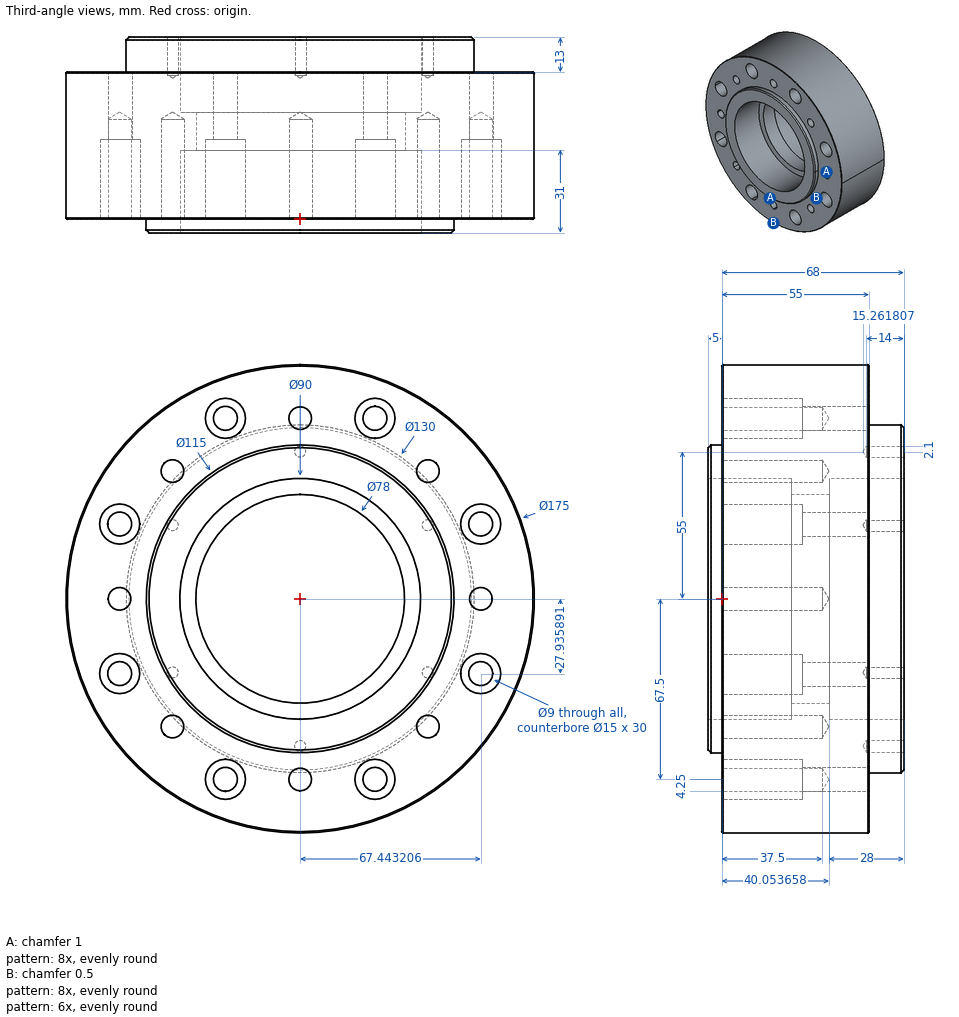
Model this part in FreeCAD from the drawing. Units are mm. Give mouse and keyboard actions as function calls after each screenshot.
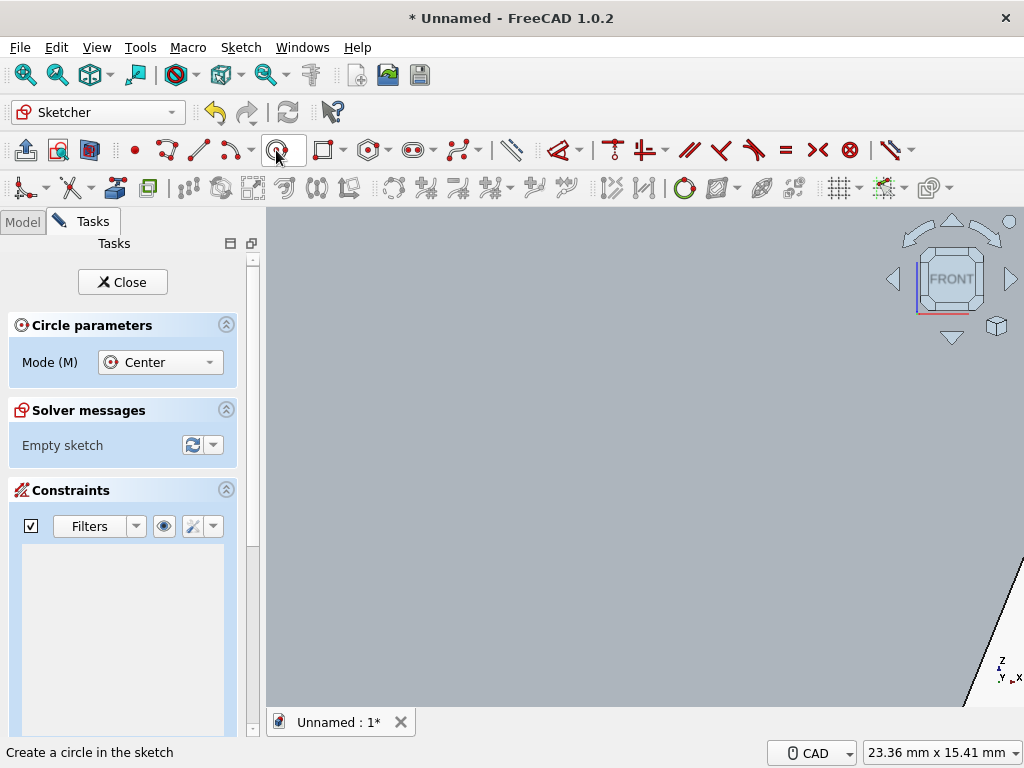
click(568, 440)
click(672, 337)
key(Escape)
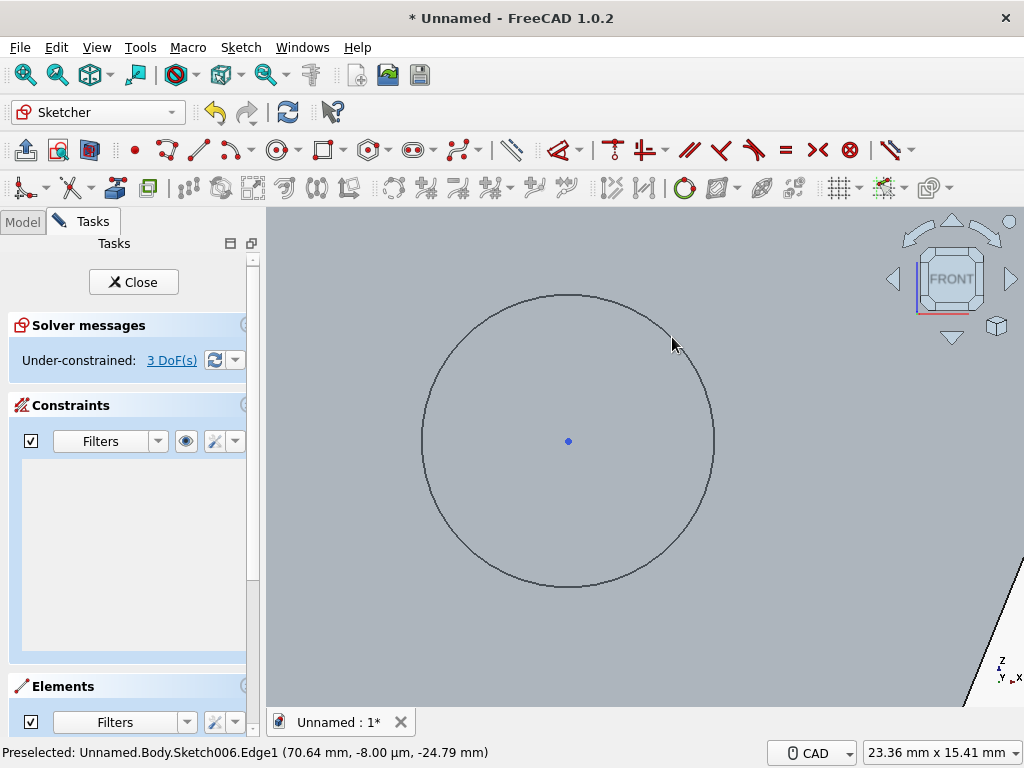
click(558, 150)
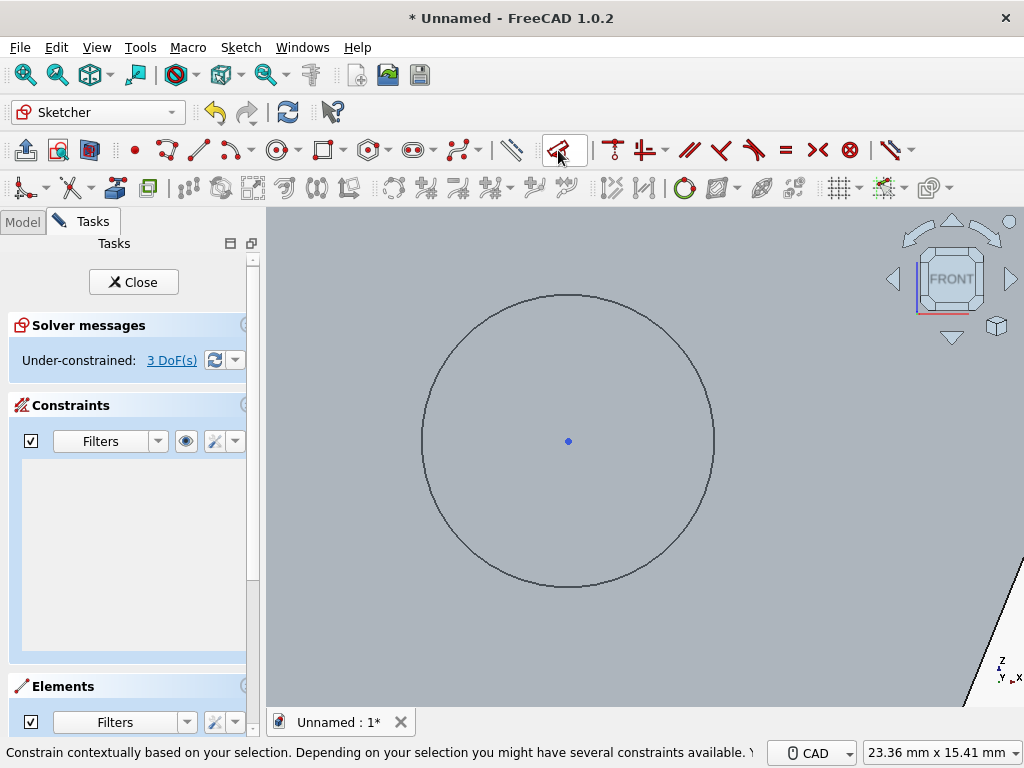
click(671, 337)
click(694, 314)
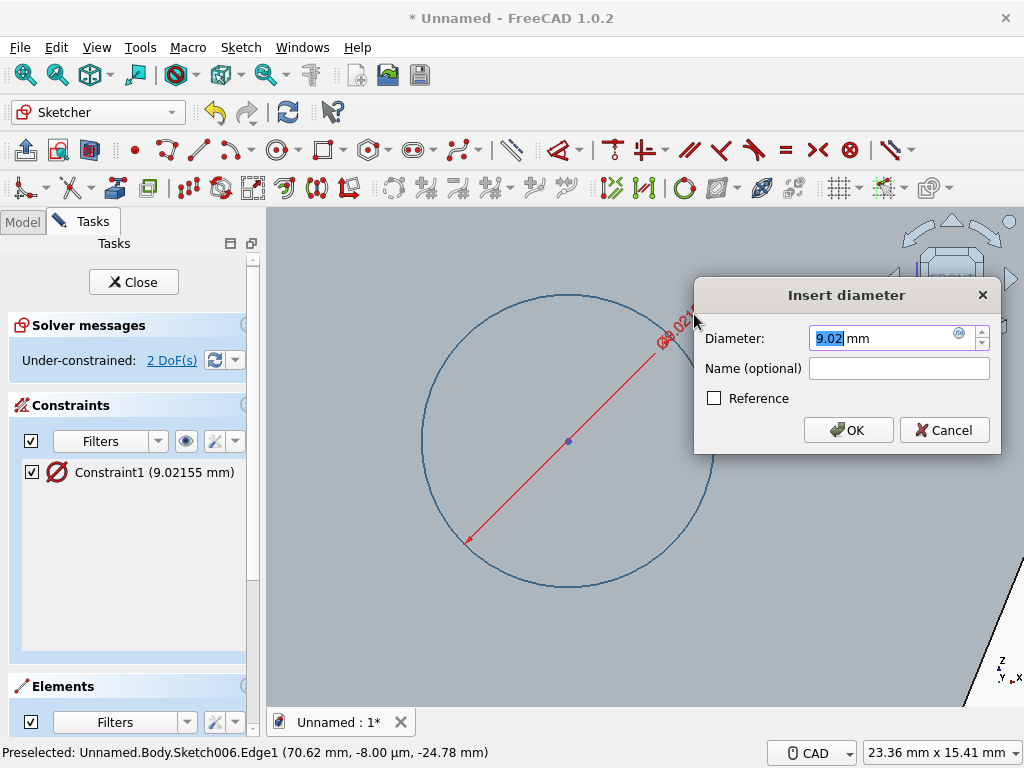
text(9)
key(Return)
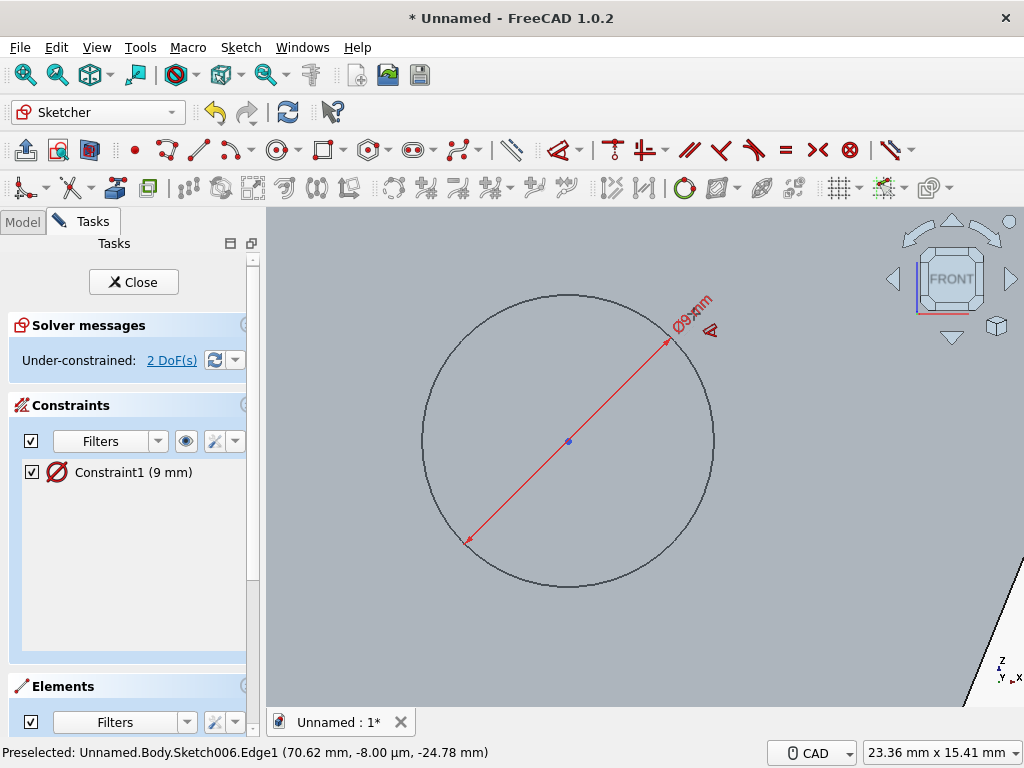
click(568, 441)
click(368, 475)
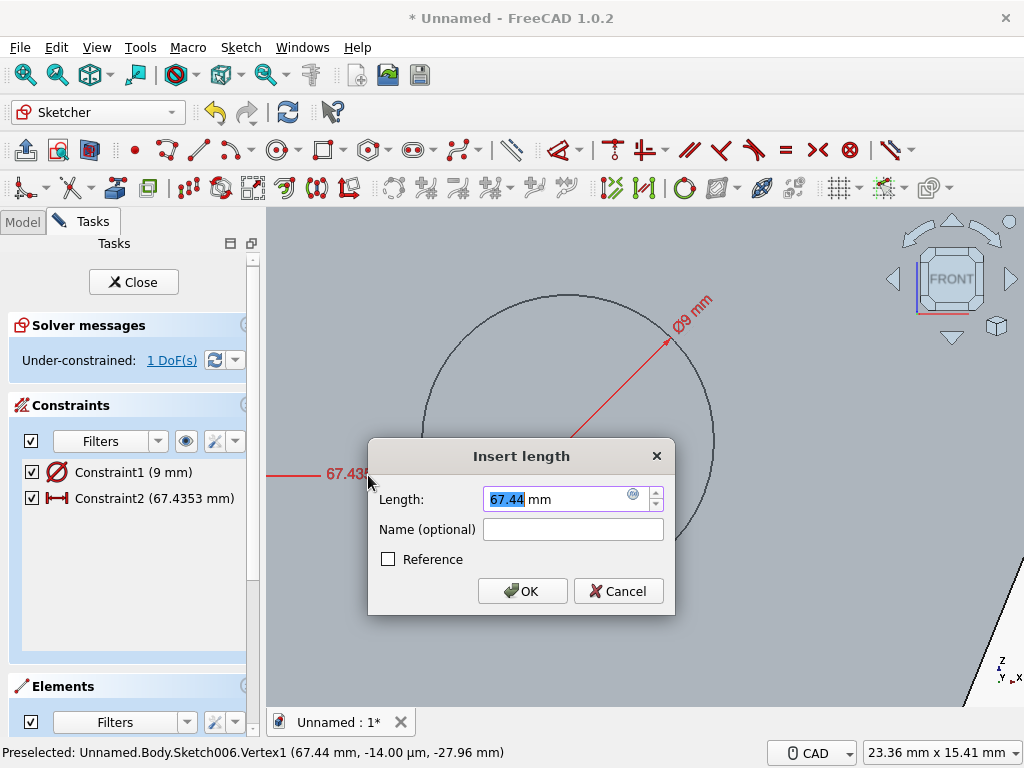
text(67.443206)
key(Return)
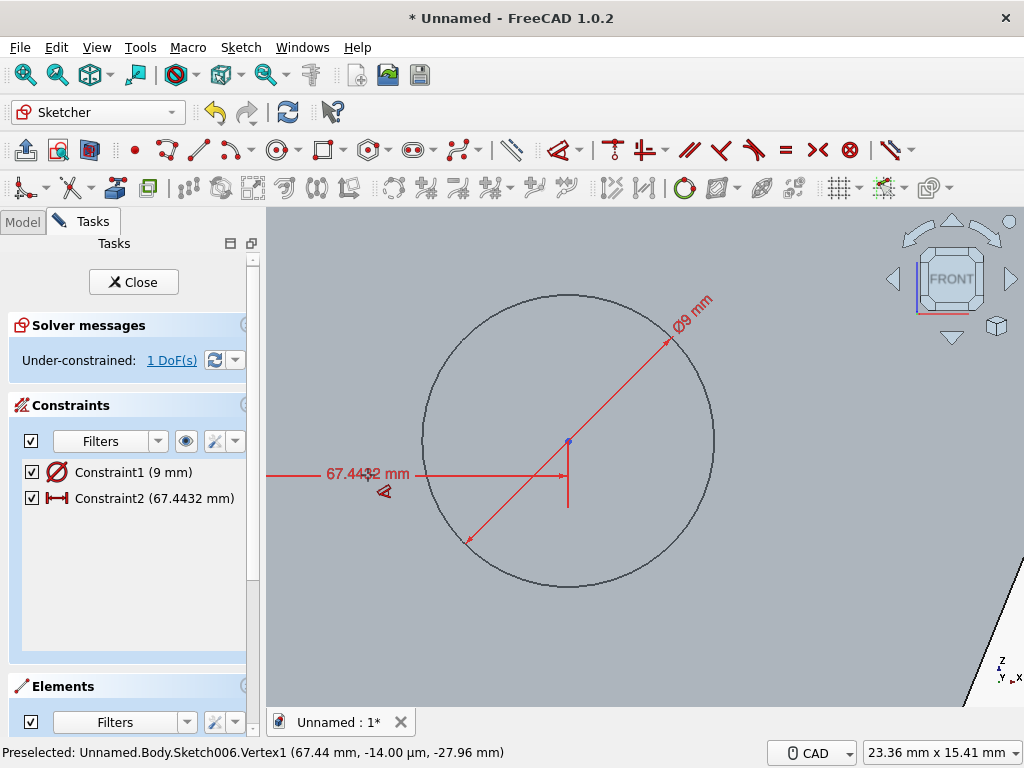
click(568, 441)
click(602, 338)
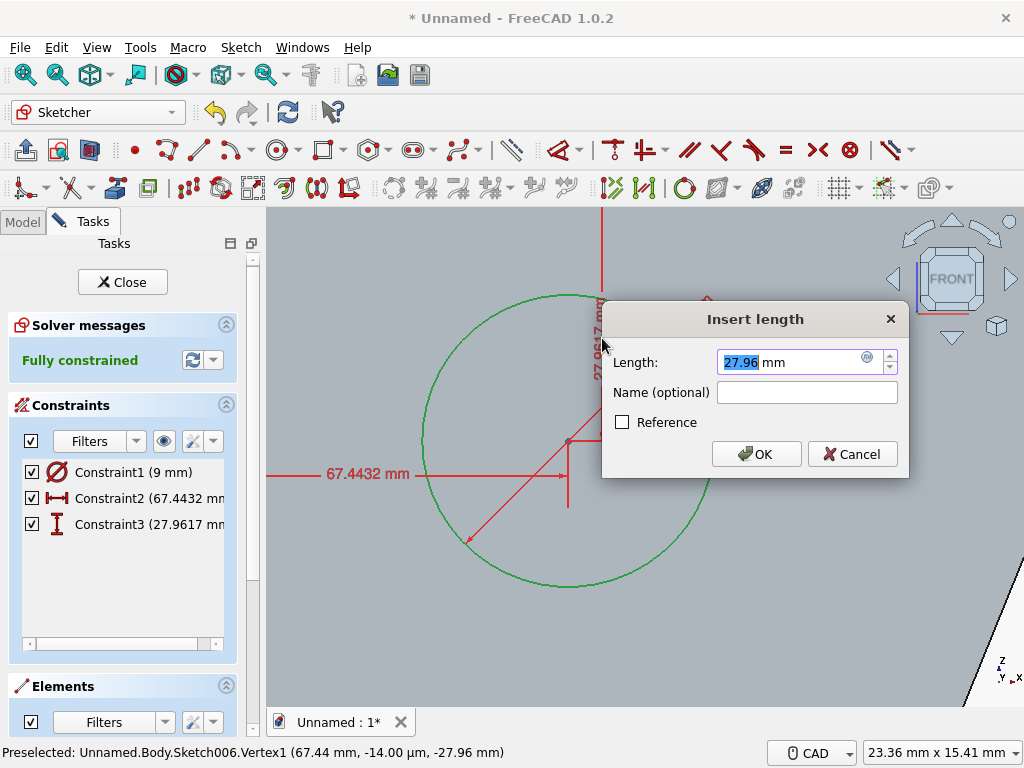
text(27.935891)
key(Return)
key(Escape)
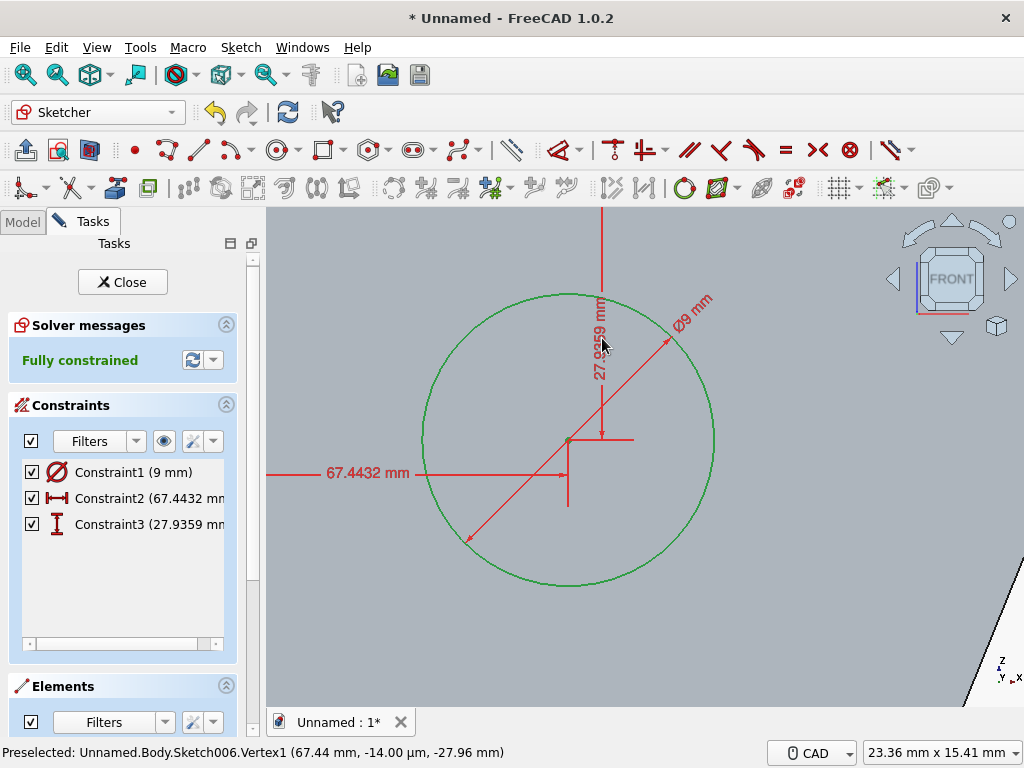
click(123, 282)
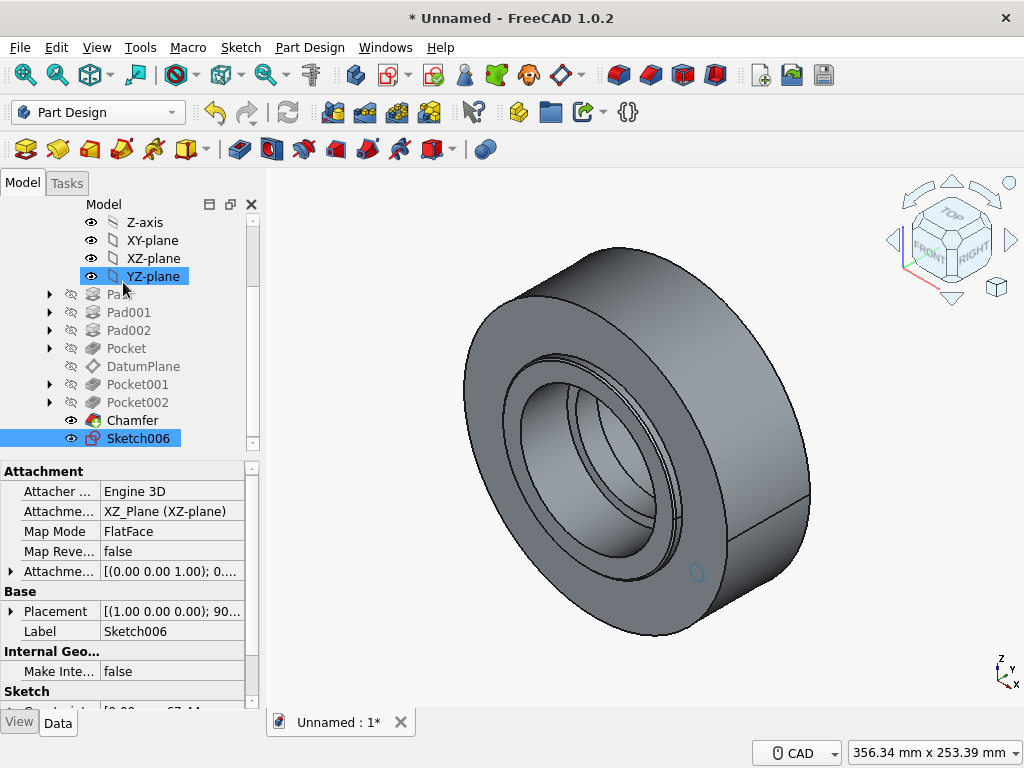
click(272, 150)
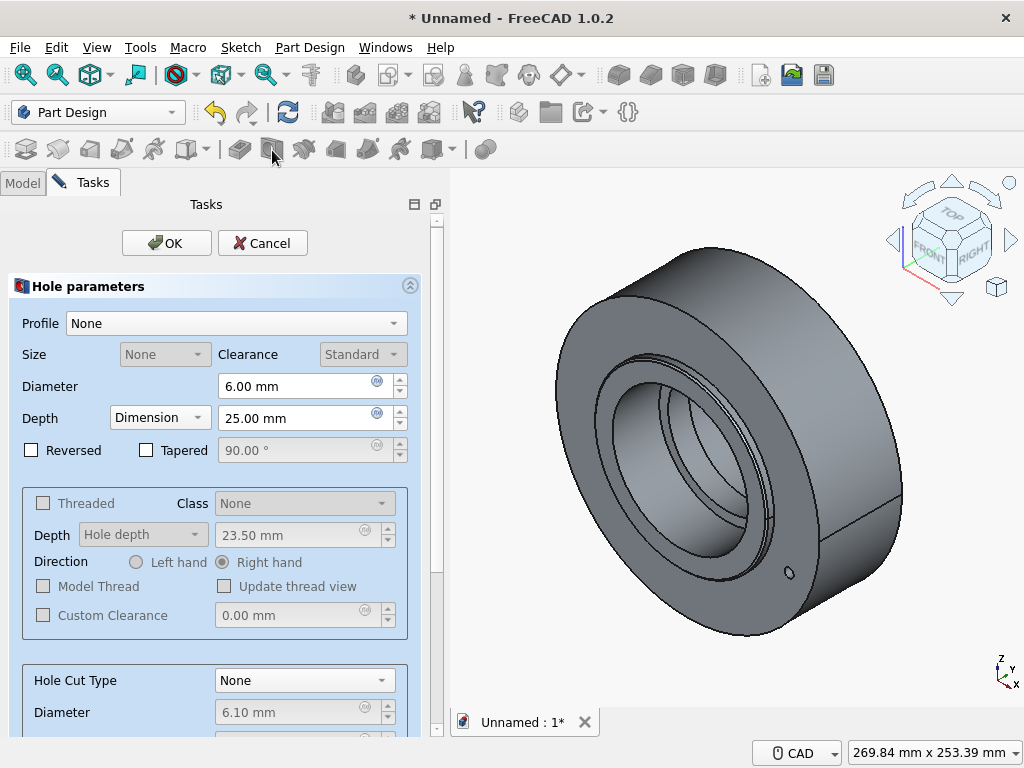
triple_click(305, 386)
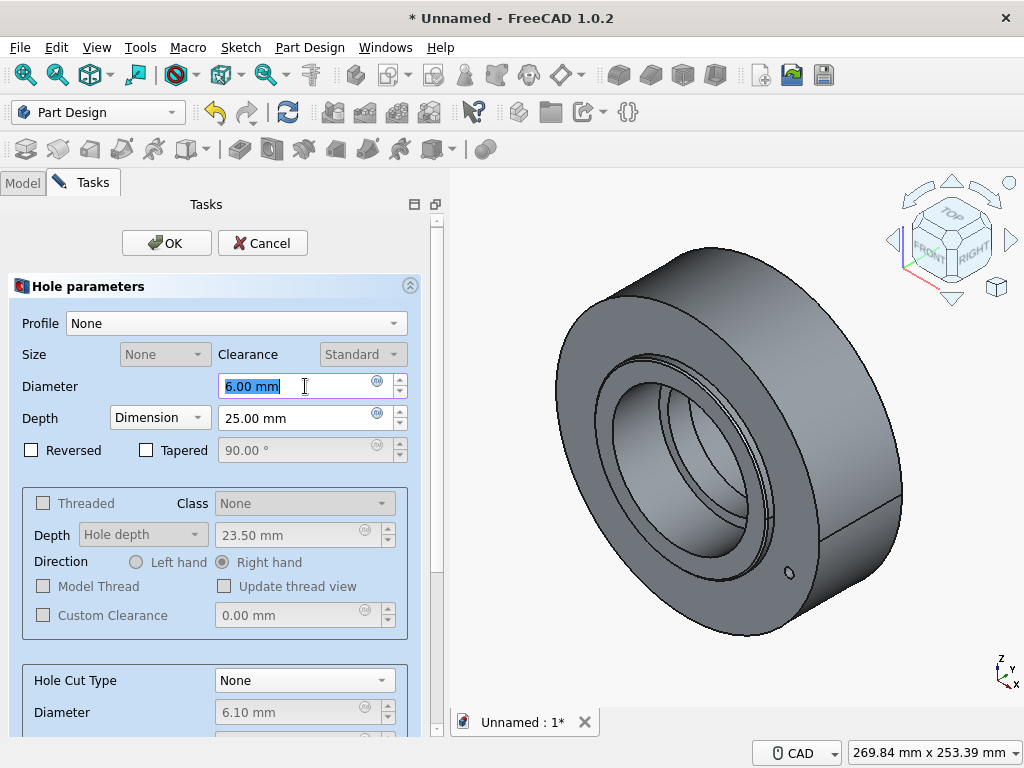
text(9)
key(Tab)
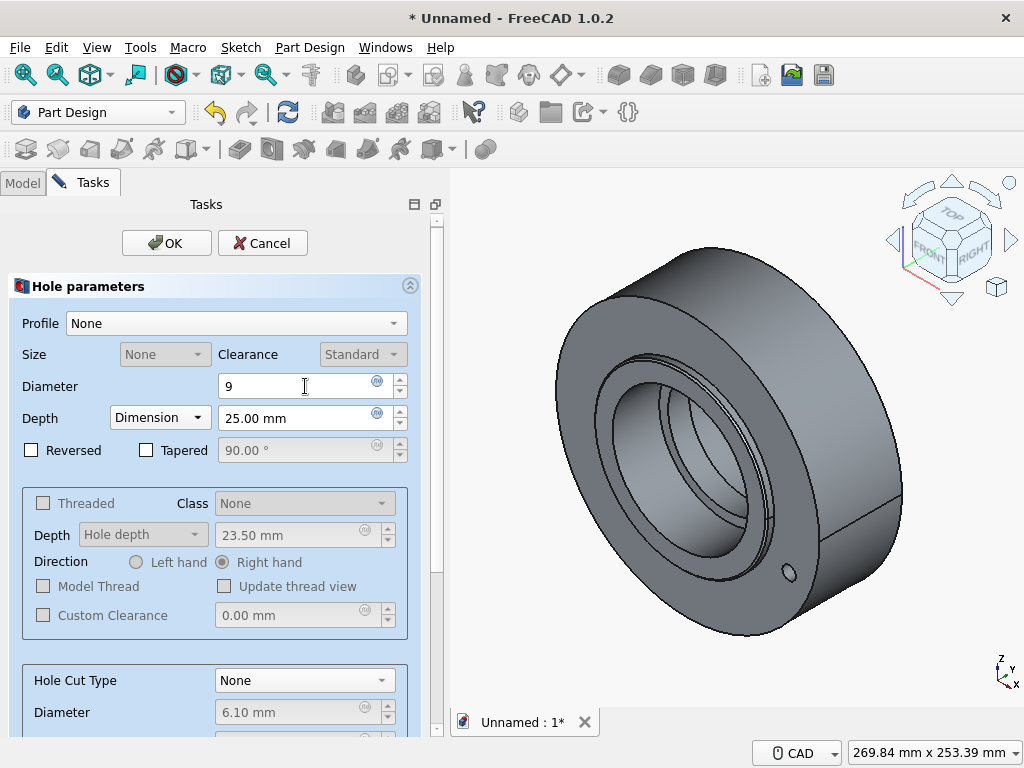
click(161, 418)